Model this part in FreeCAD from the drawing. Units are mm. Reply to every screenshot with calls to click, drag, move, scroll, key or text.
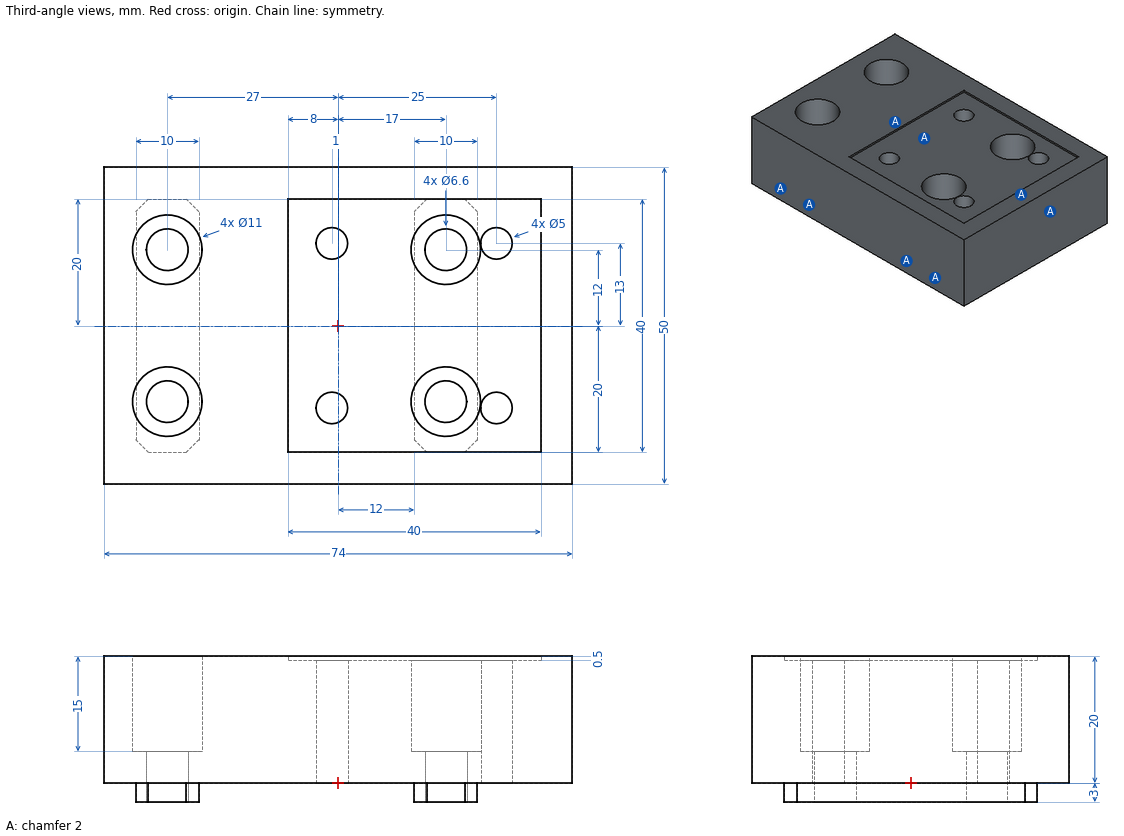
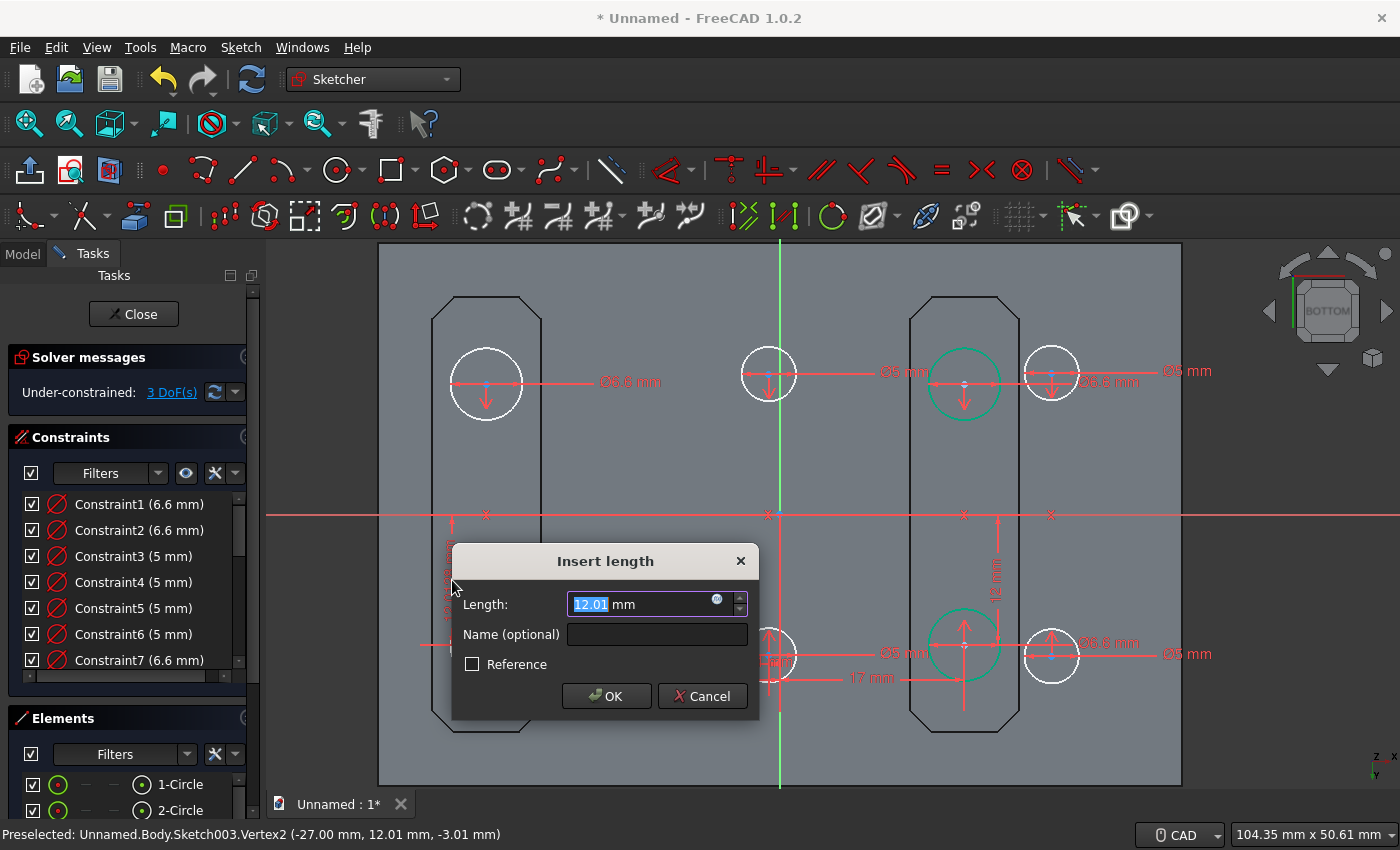
text(12)
key(Return)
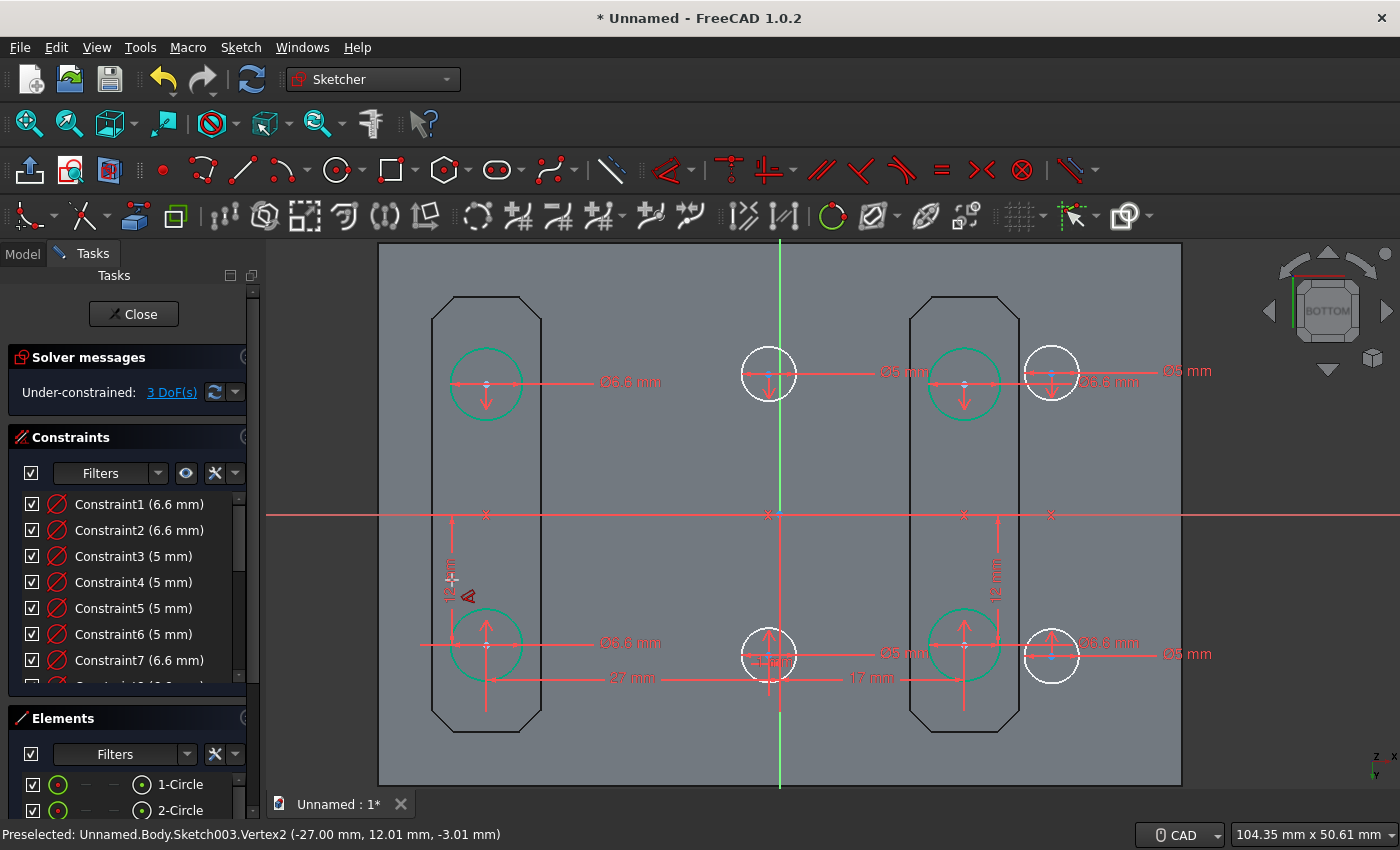
click(1052, 656)
click(1011, 690)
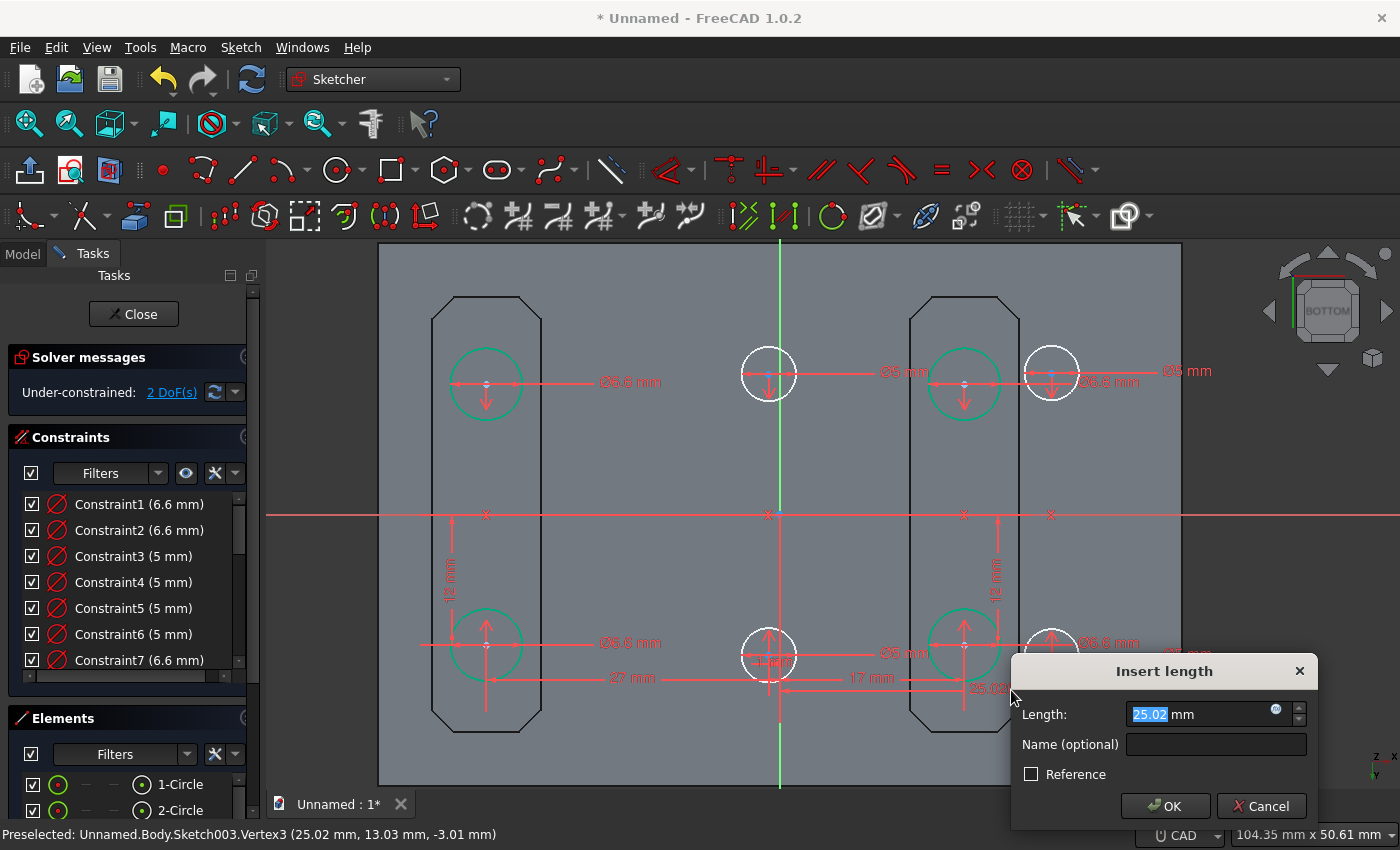
text(25)
key(Return)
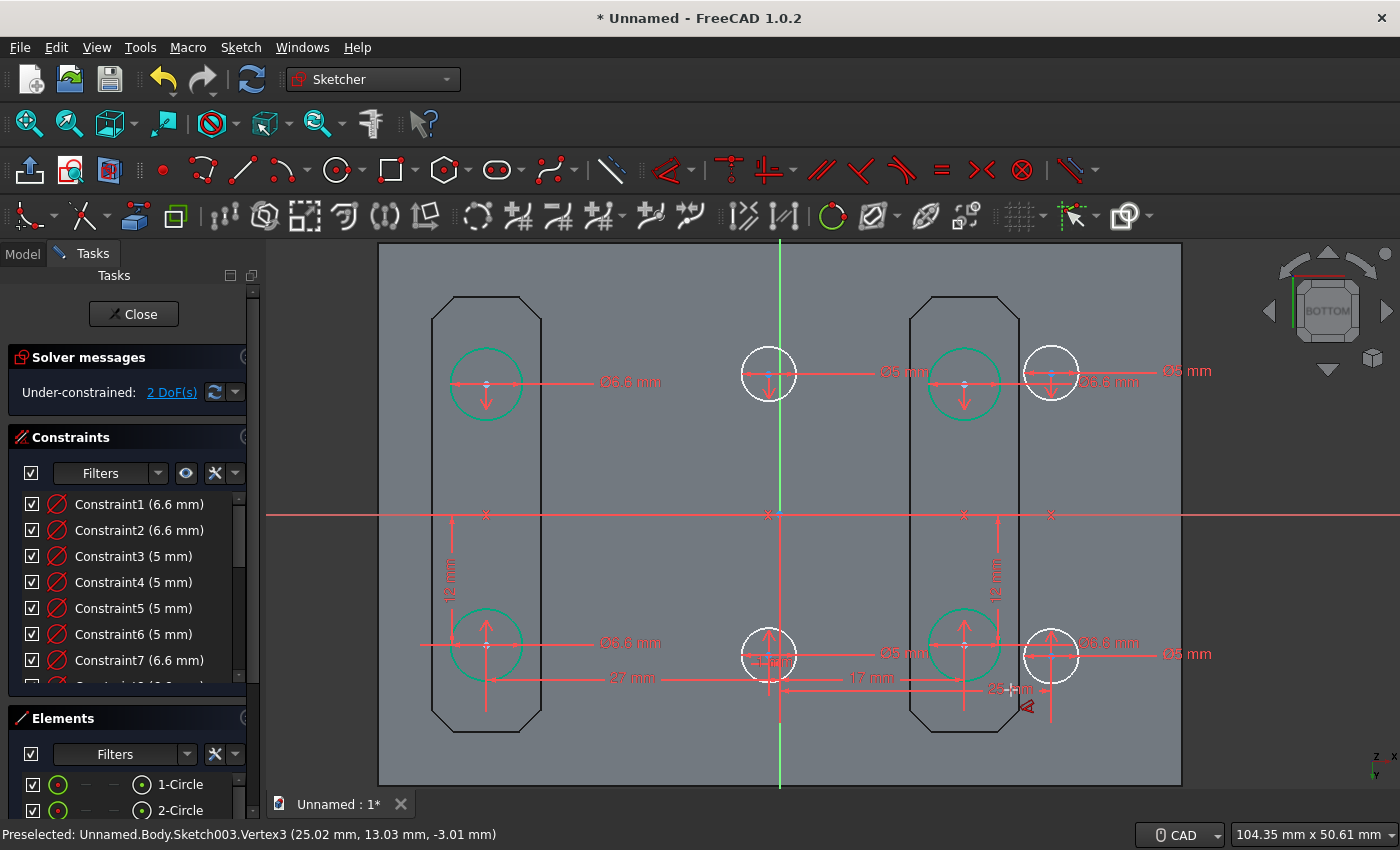
click(1051, 656)
click(1085, 585)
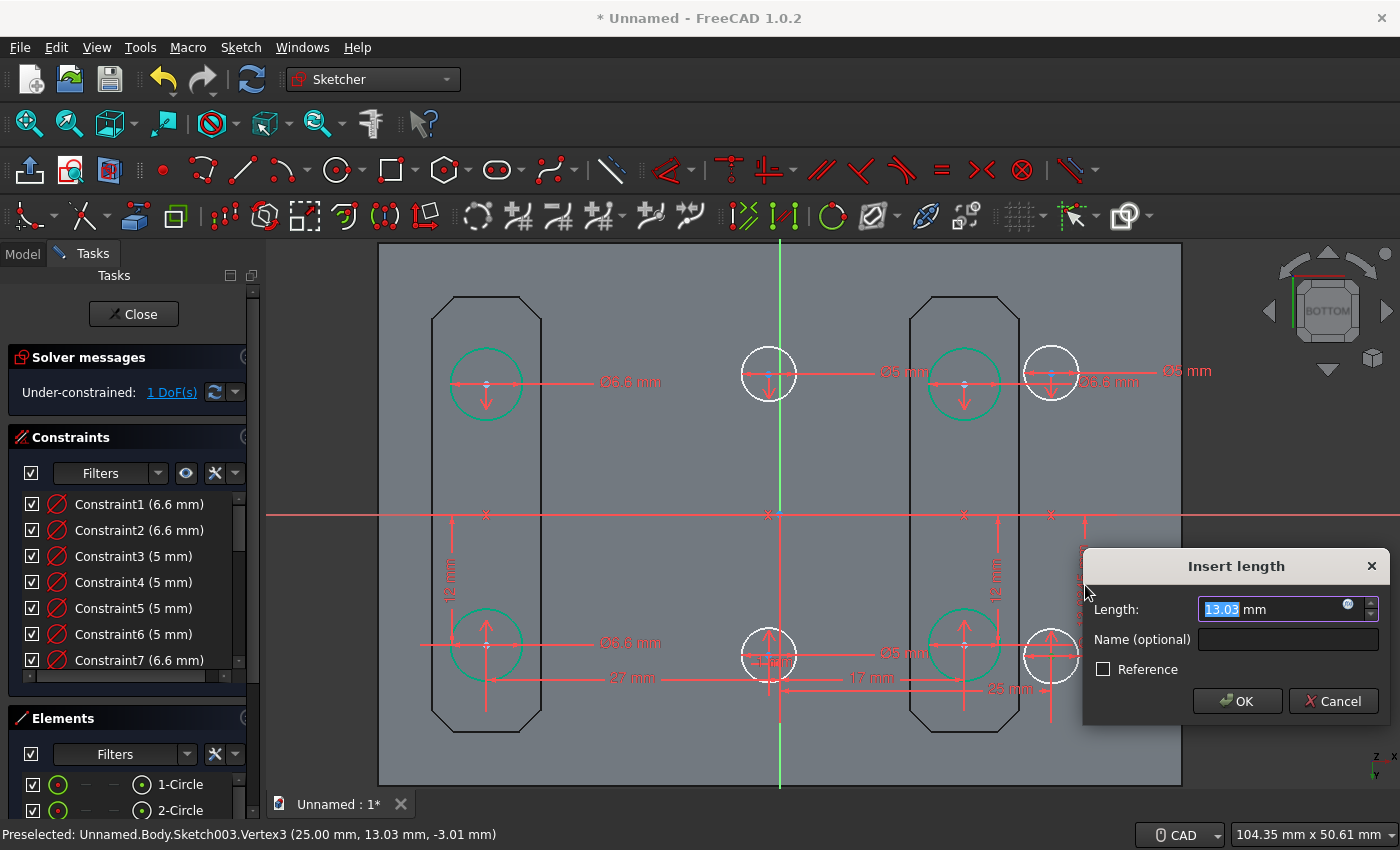
text(13)
key(Return)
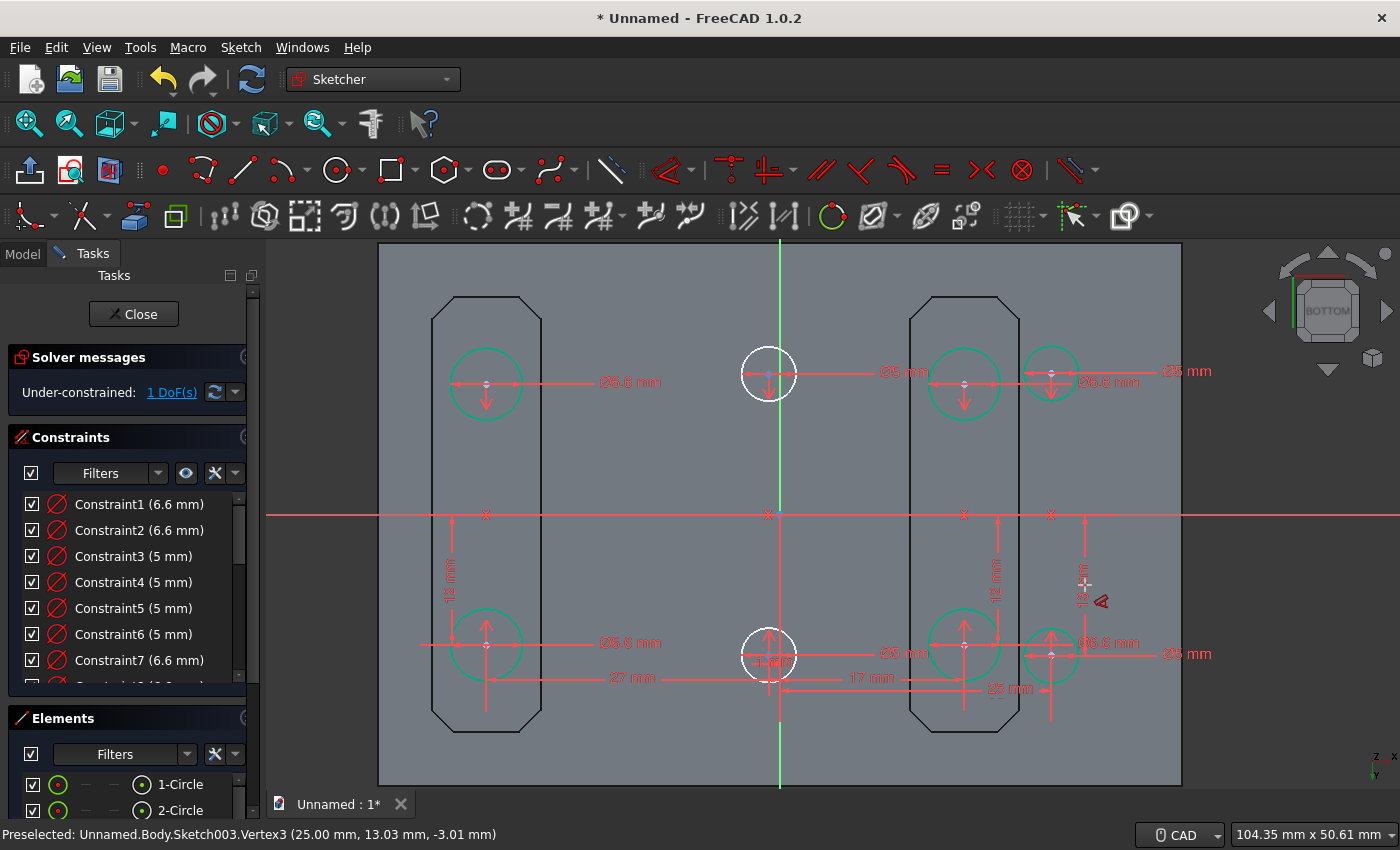
click(769, 655)
click(814, 585)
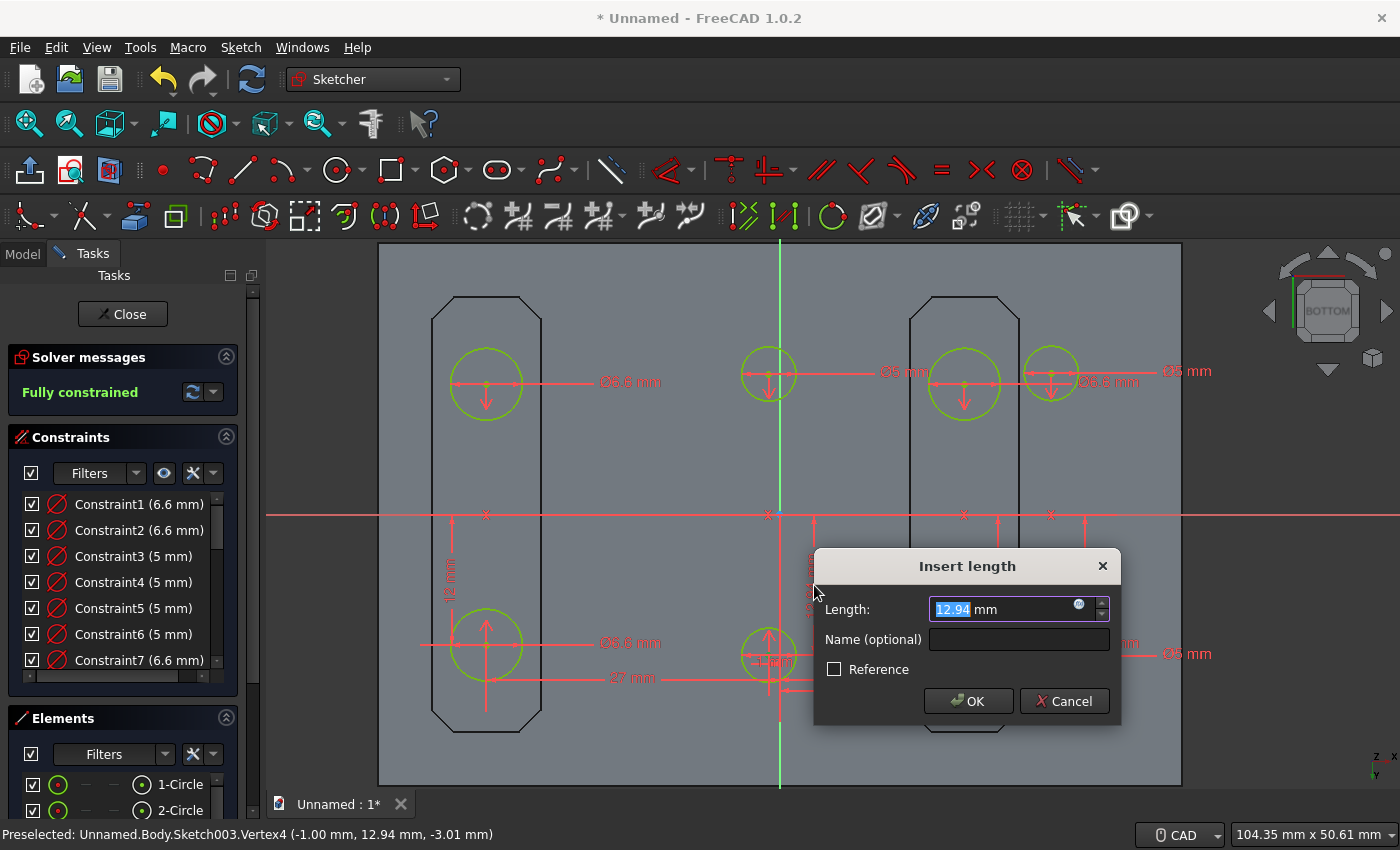
text(13)
key(Return)
key(Escape)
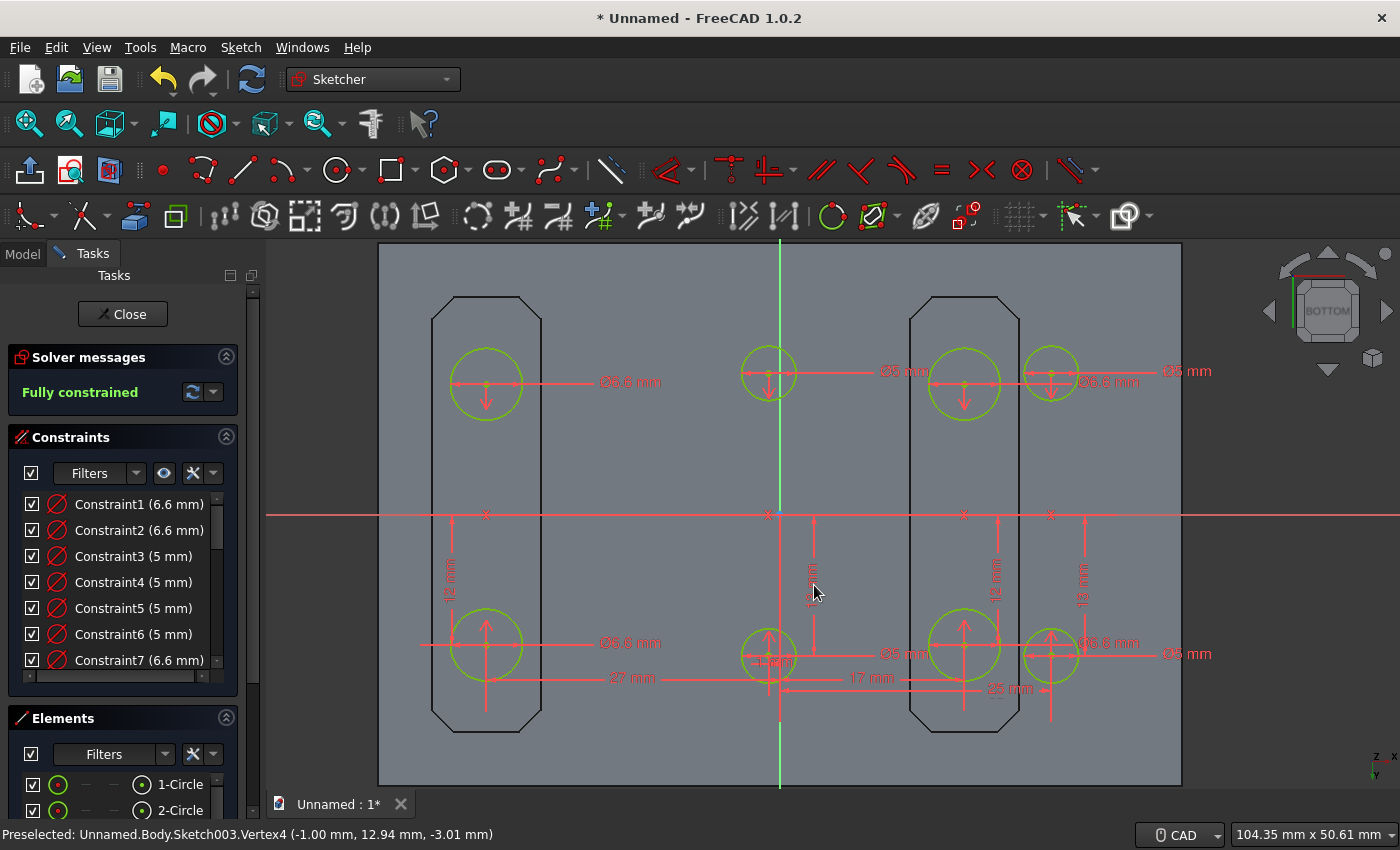
click(123, 314)